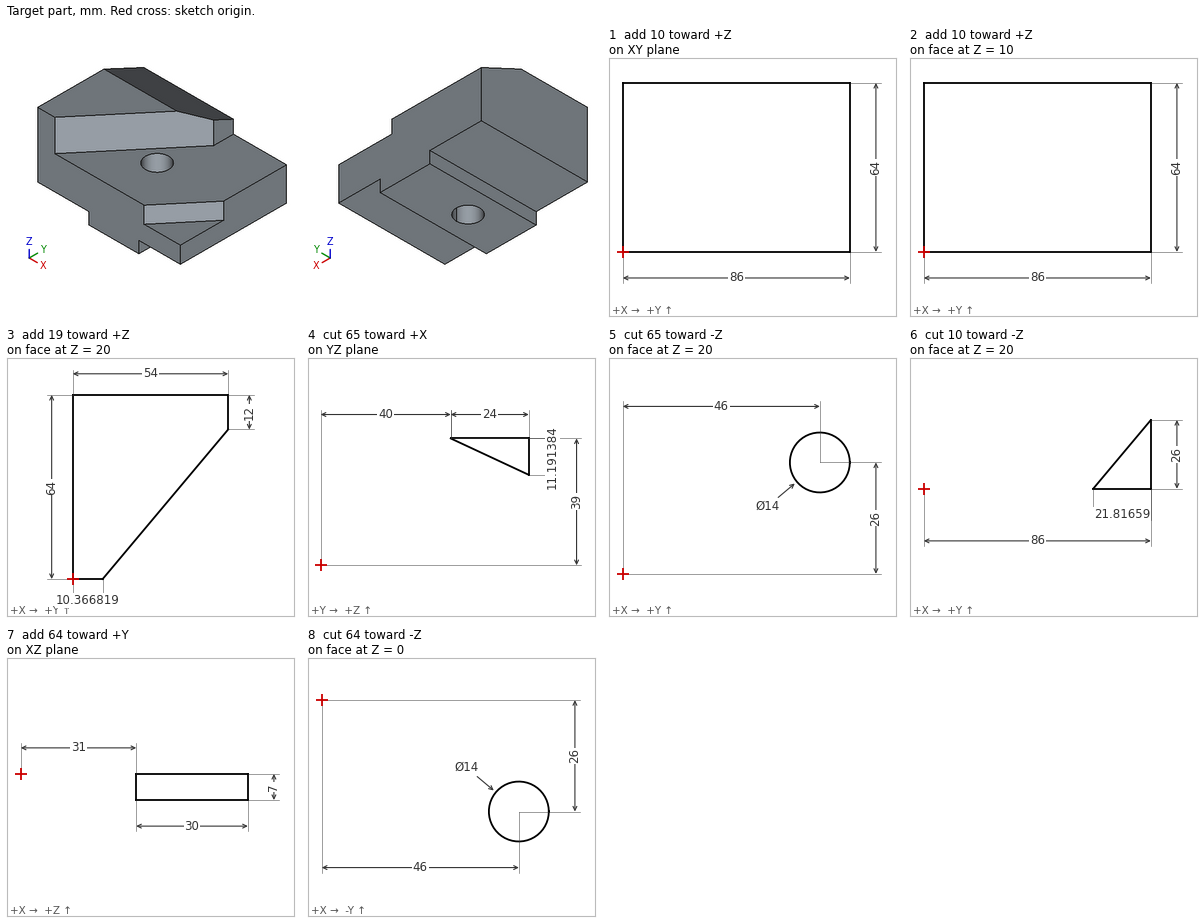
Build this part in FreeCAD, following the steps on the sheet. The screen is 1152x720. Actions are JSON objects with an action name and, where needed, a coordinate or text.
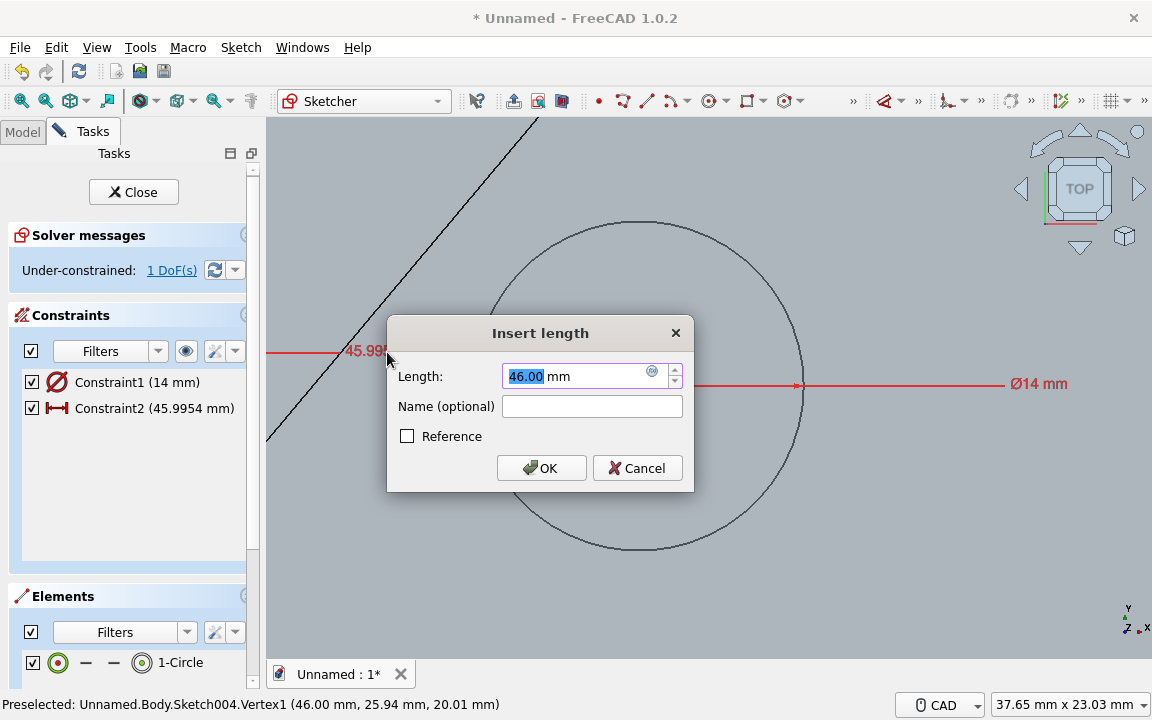
{"action": "type", "text": "46"}
{"action": "key", "text": "Return"}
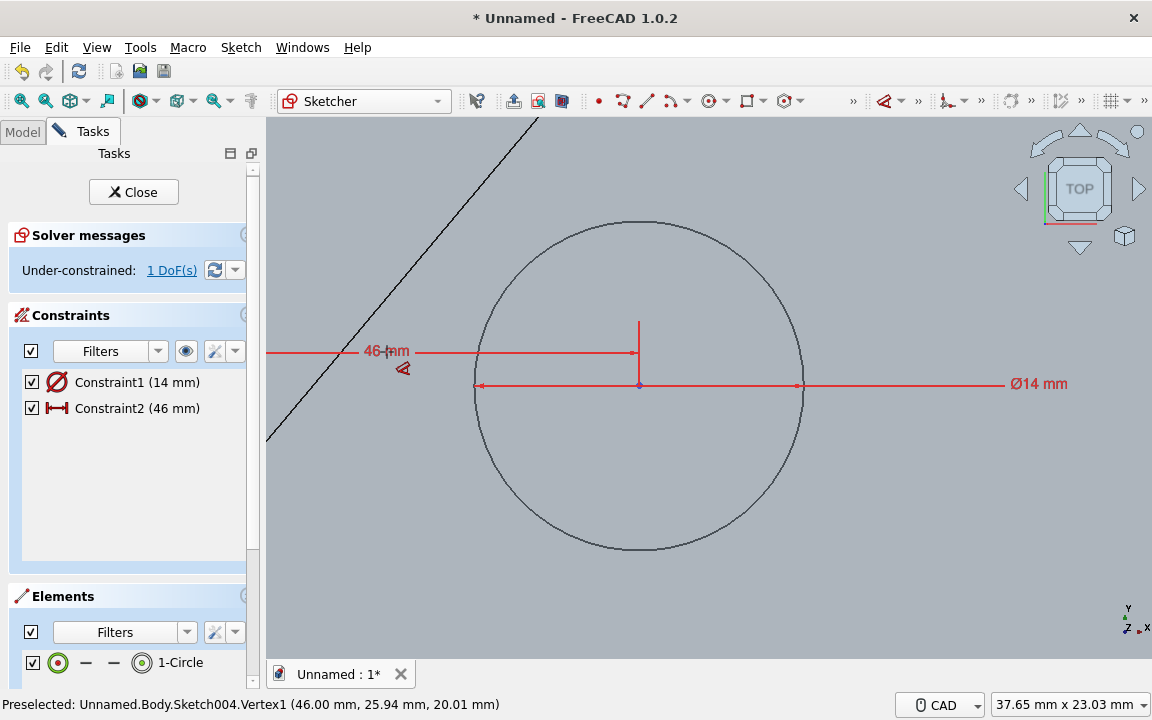
{"action": "left_click", "coordinate": [639, 386]}
{"action": "left_click", "coordinate": [673, 508]}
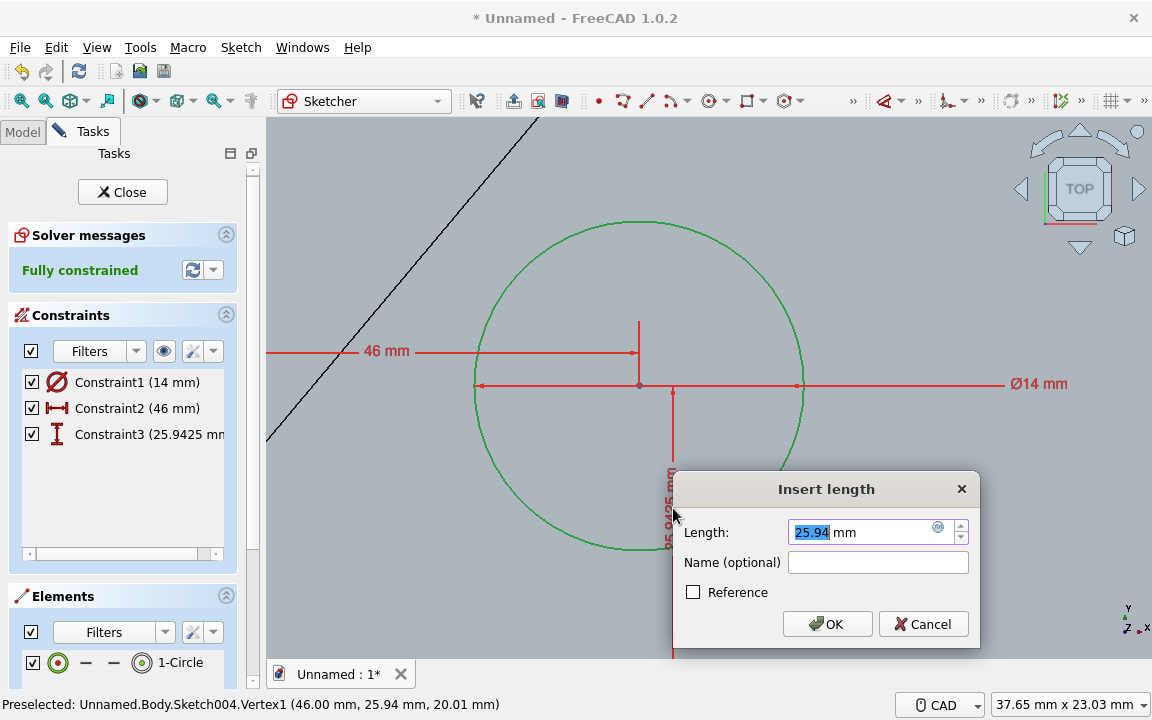
{"action": "type", "text": "26"}
{"action": "key", "text": "Return"}
{"action": "key", "text": "Escape"}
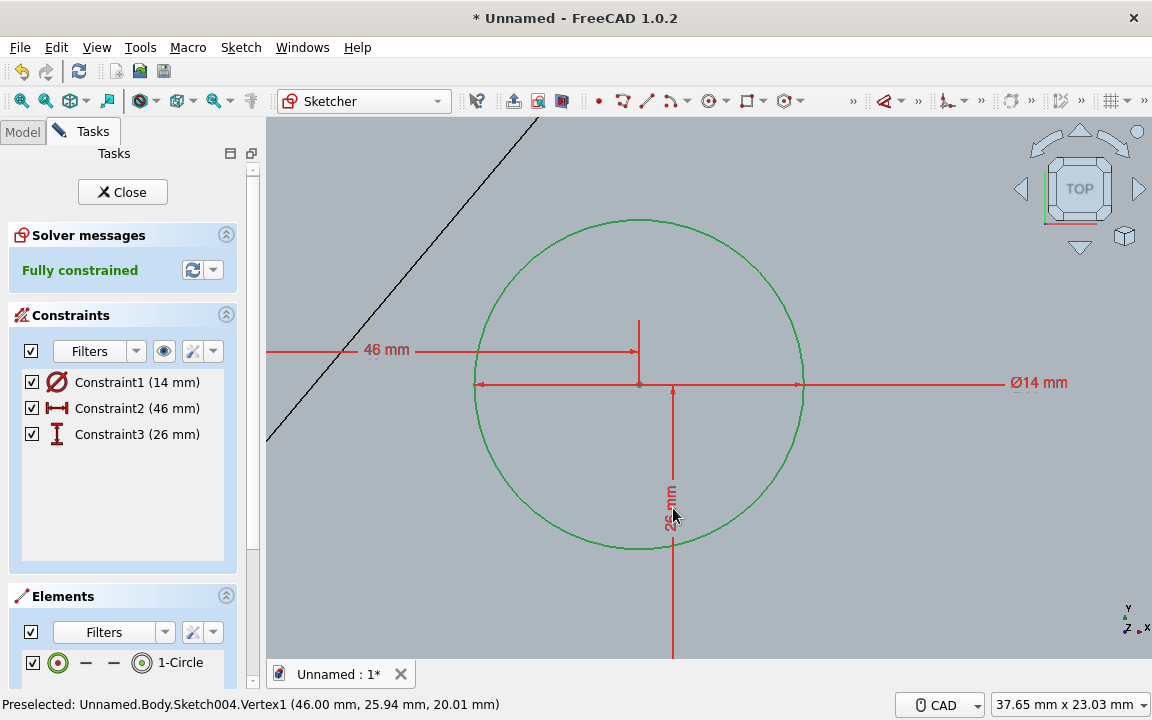
{"action": "left_click", "coordinate": [123, 192]}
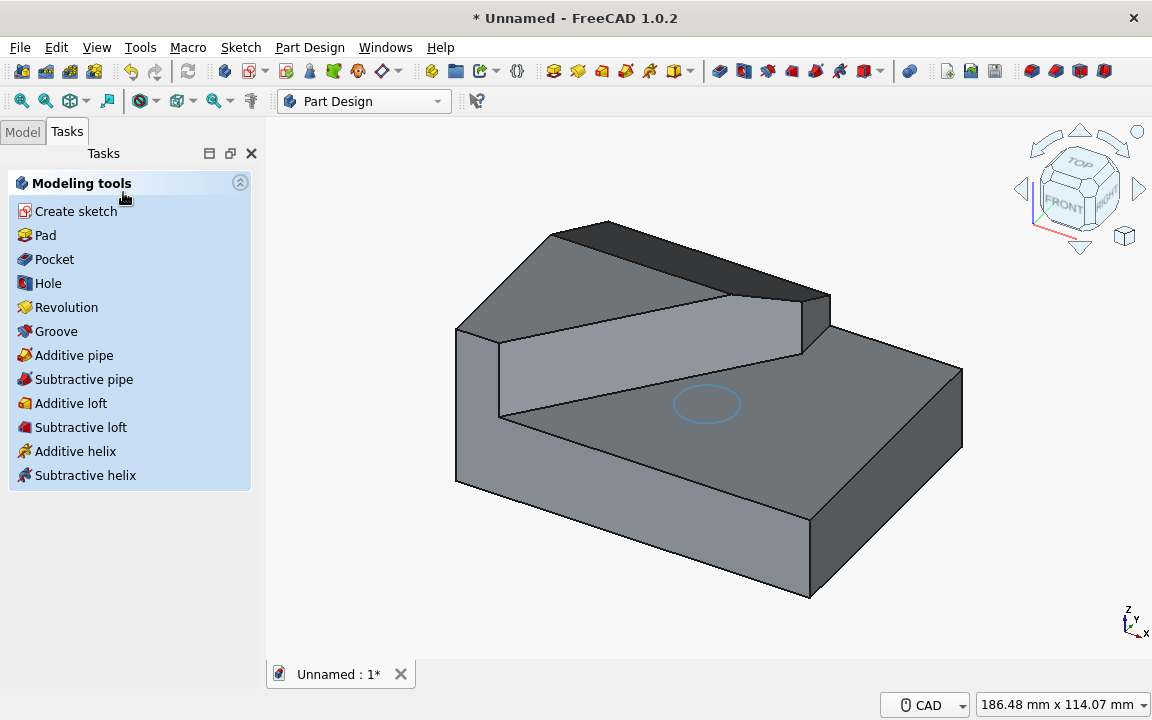
{"action": "left_click", "coordinate": [720, 72]}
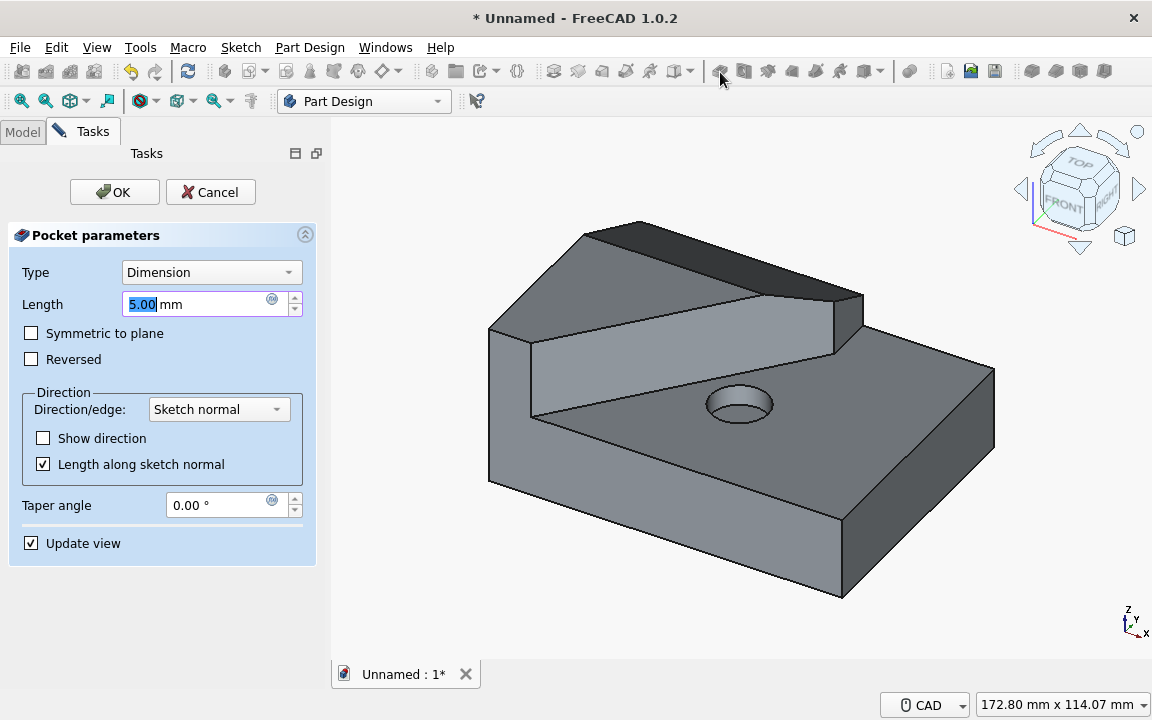
{"action": "type", "text": "65"}
{"action": "key", "text": "Tab"}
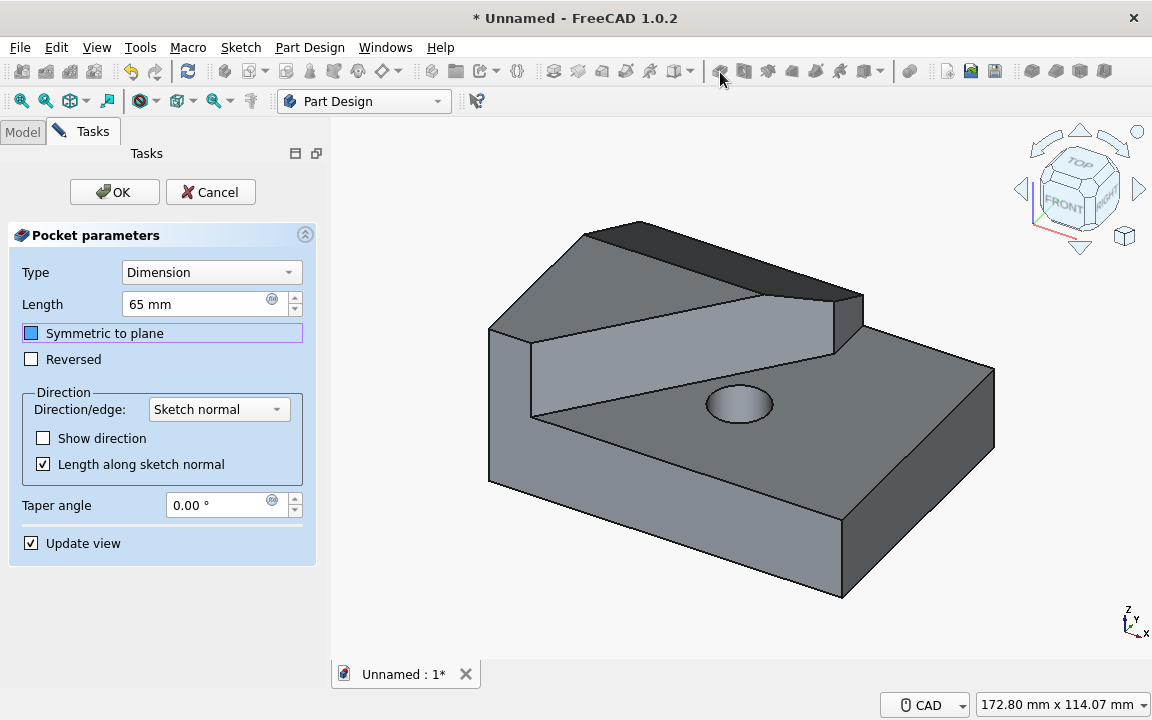
{"action": "left_click", "coordinate": [115, 192]}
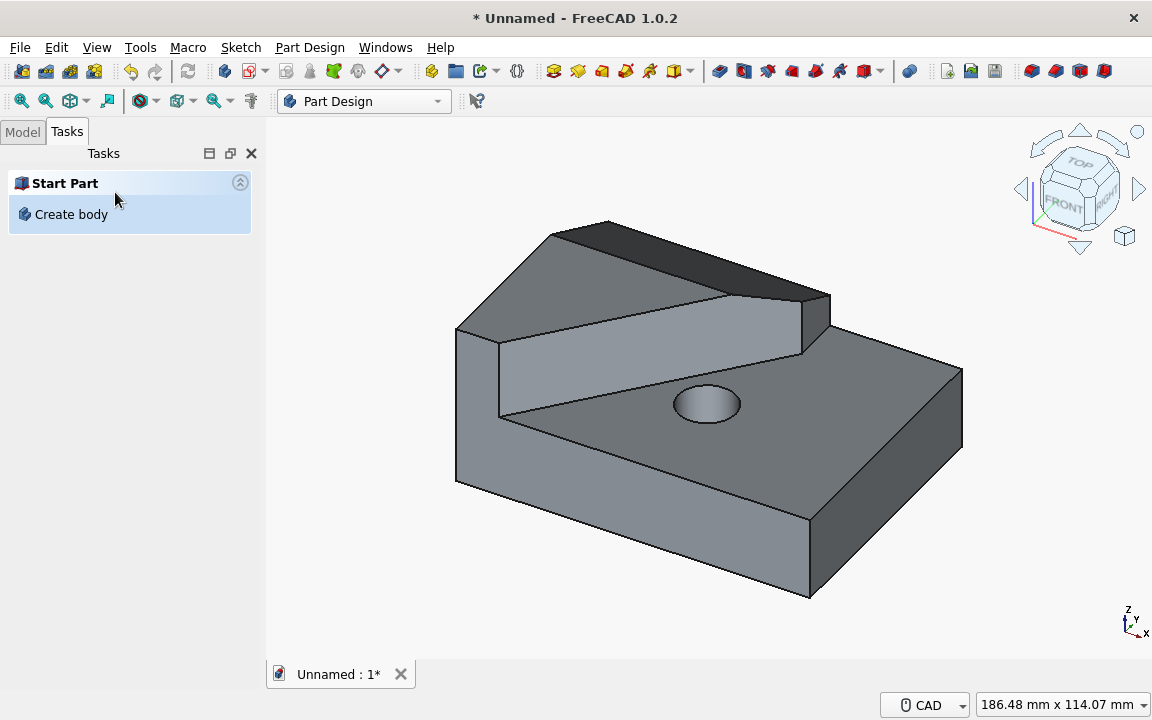
{"action": "left_click", "coordinate": [841, 400]}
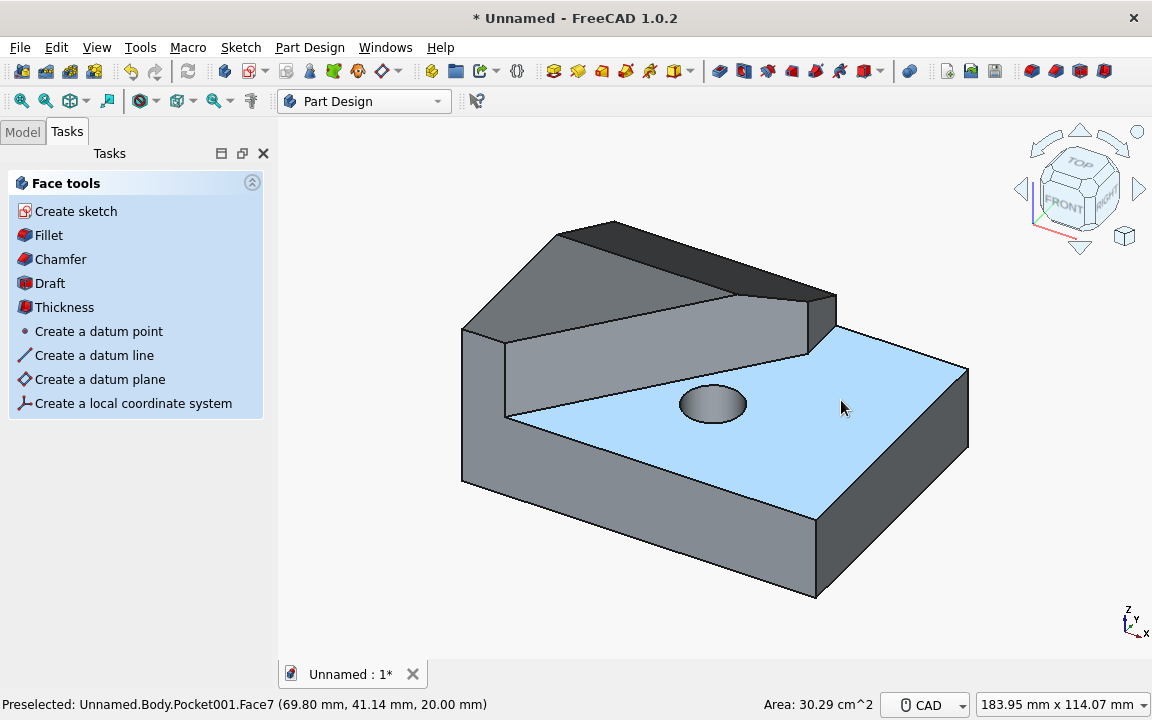
{"action": "left_click", "coordinate": [250, 72]}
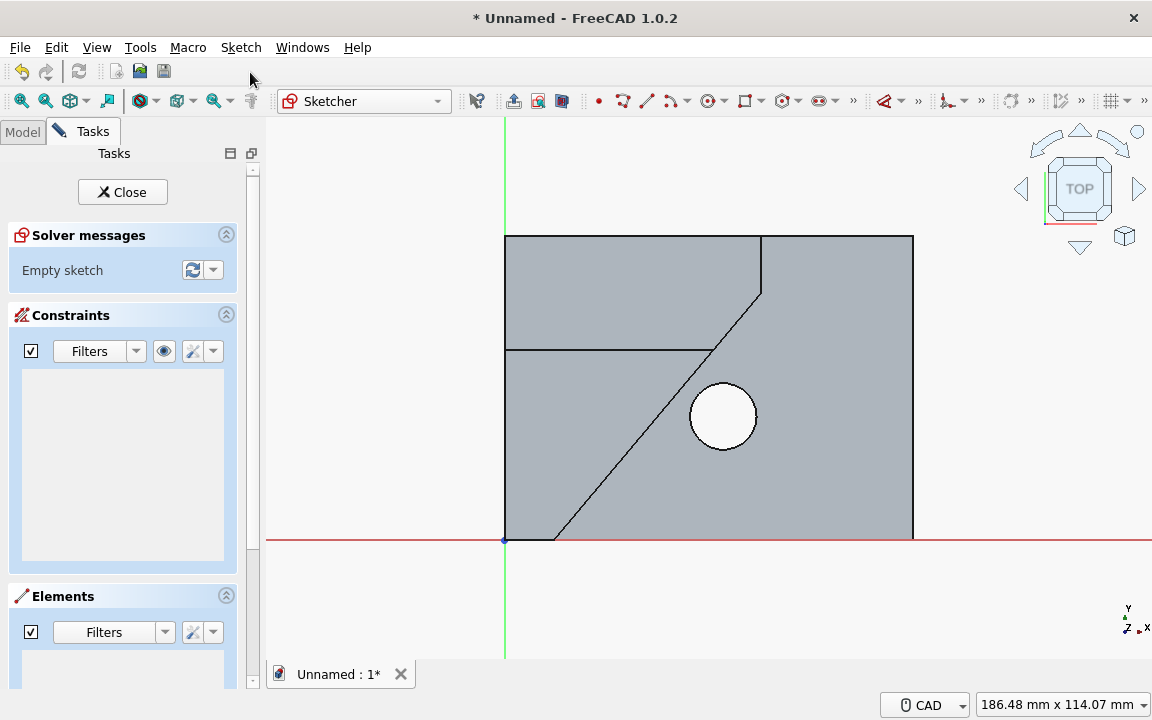
{"action": "left_click", "coordinate": [562, 102]}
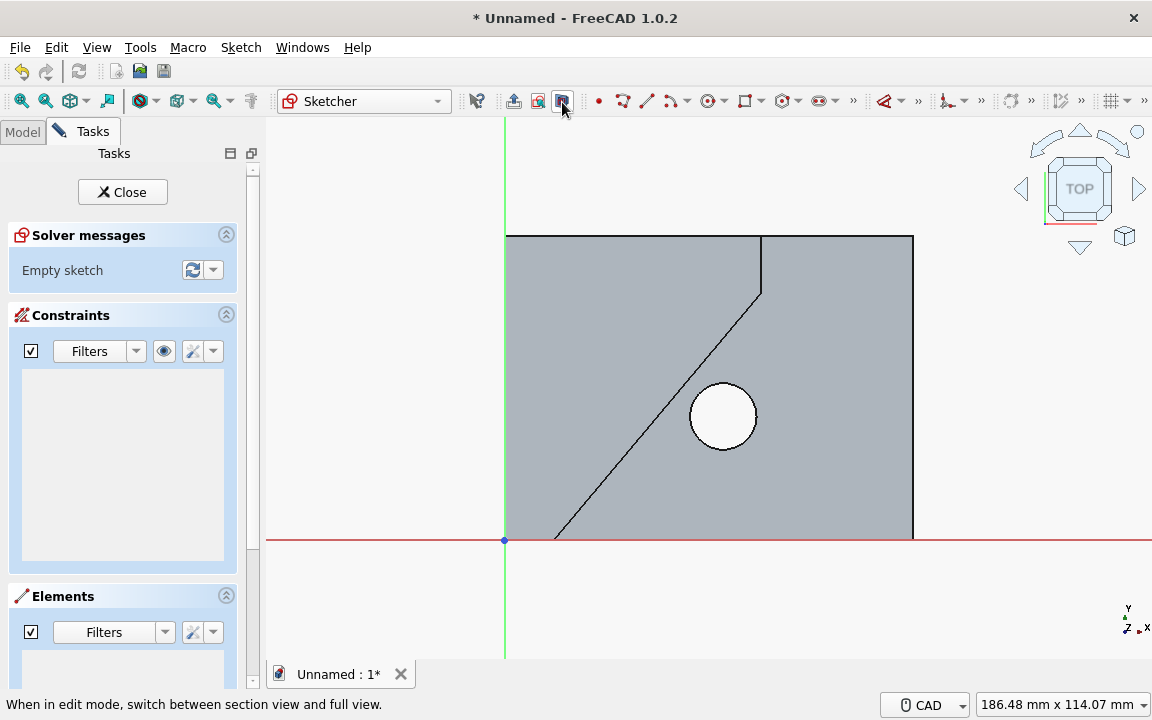
{"action": "scroll", "coordinate": [987, 531], "scroll_direction": "up", "scroll_amount": 5}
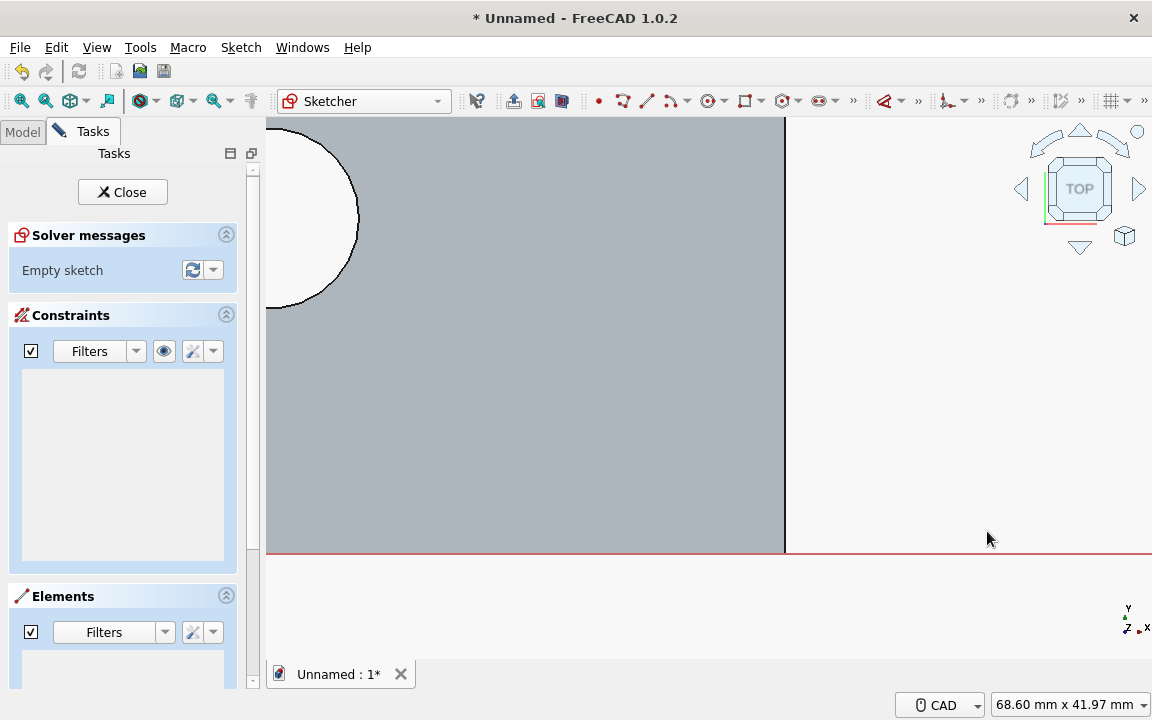
{"action": "left_click", "coordinate": [624, 102]}